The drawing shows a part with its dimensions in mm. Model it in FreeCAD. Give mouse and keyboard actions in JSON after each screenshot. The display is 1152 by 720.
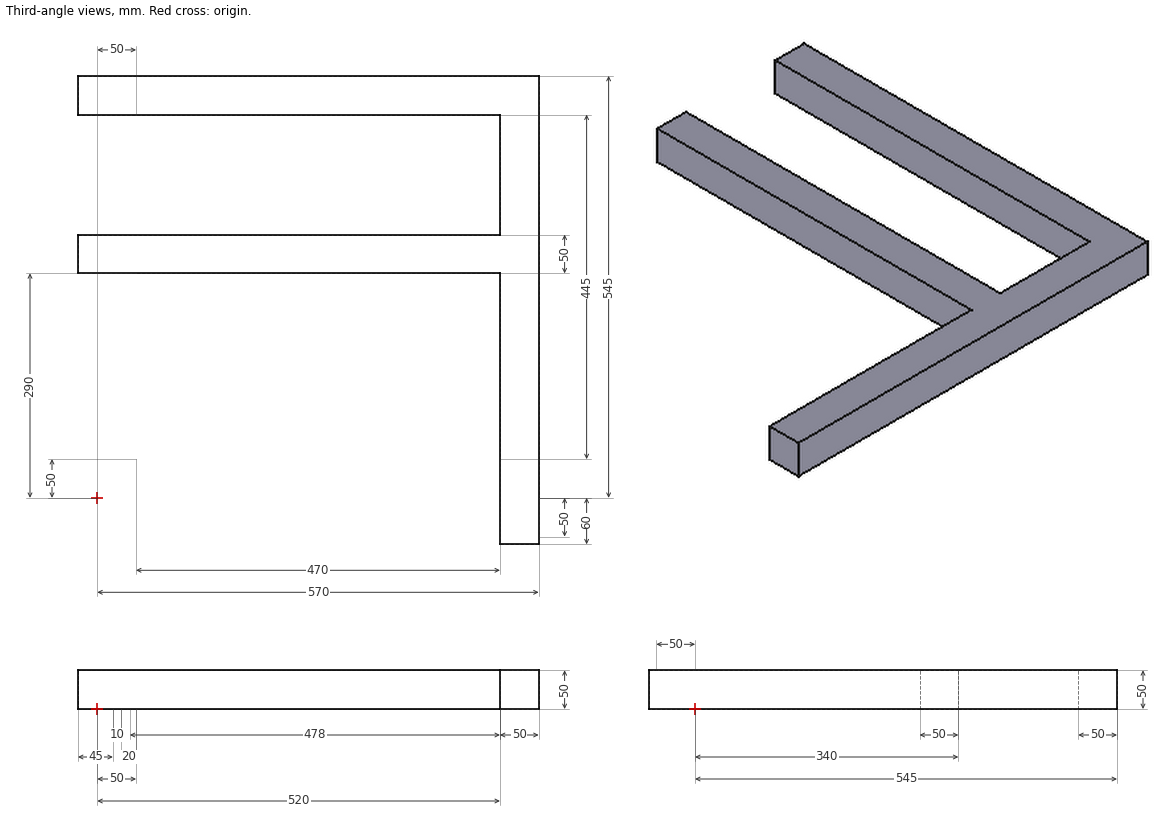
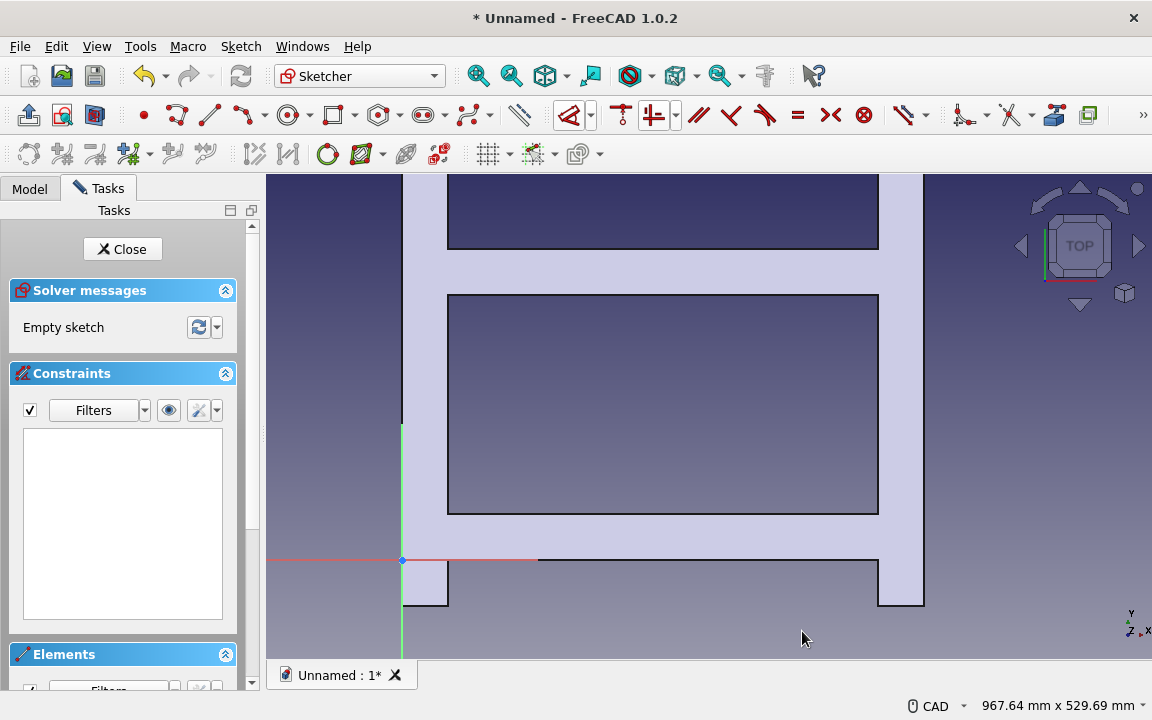
{"action": "left_click", "coordinate": [332, 116]}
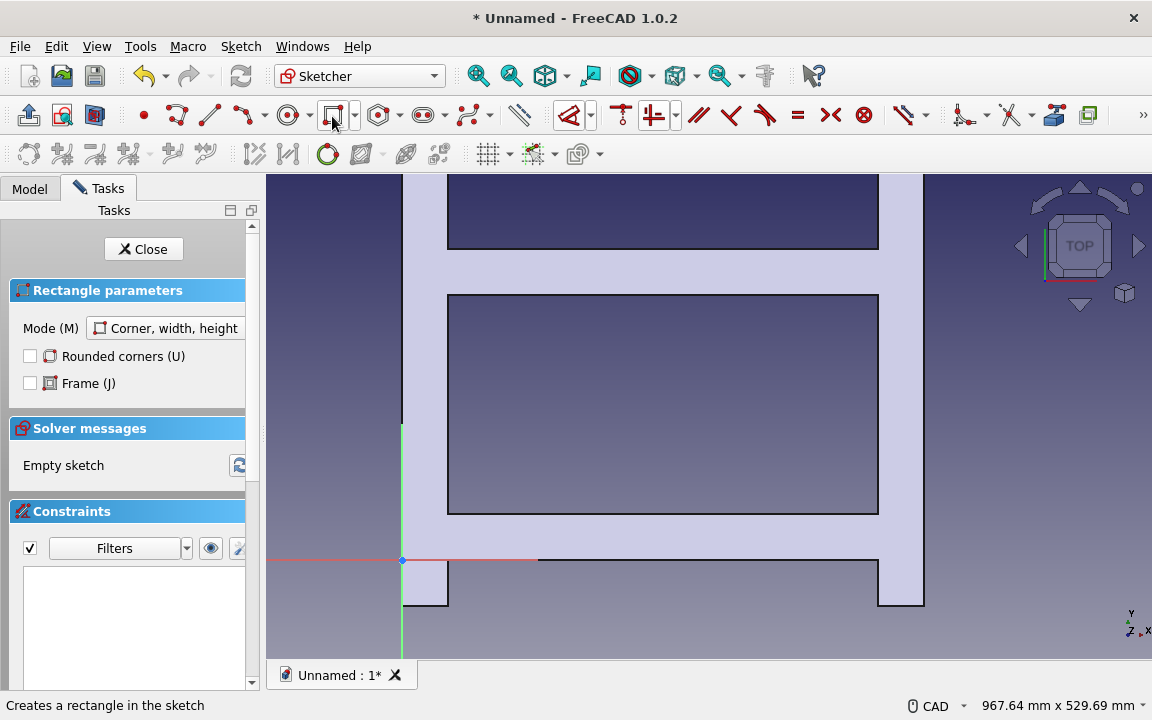
{"action": "left_click", "coordinate": [448, 514]}
{"action": "left_click", "coordinate": [878, 560]}
{"action": "key", "text": "Escape"}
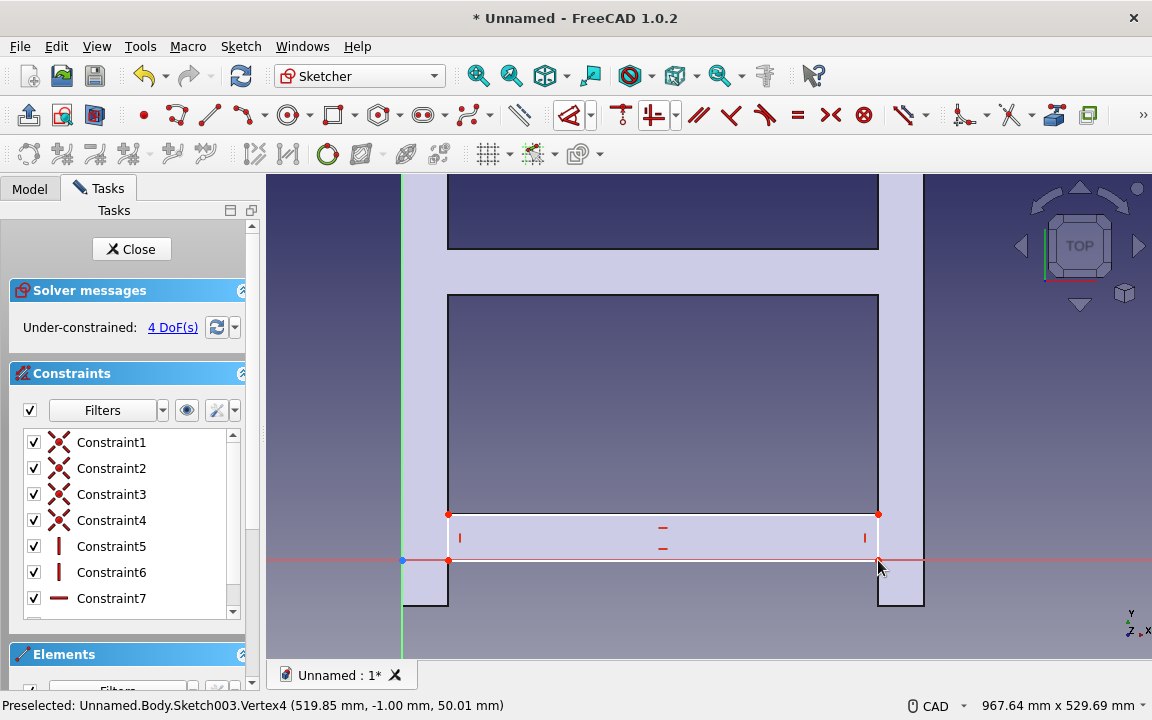
{"action": "left_click", "coordinate": [448, 561]}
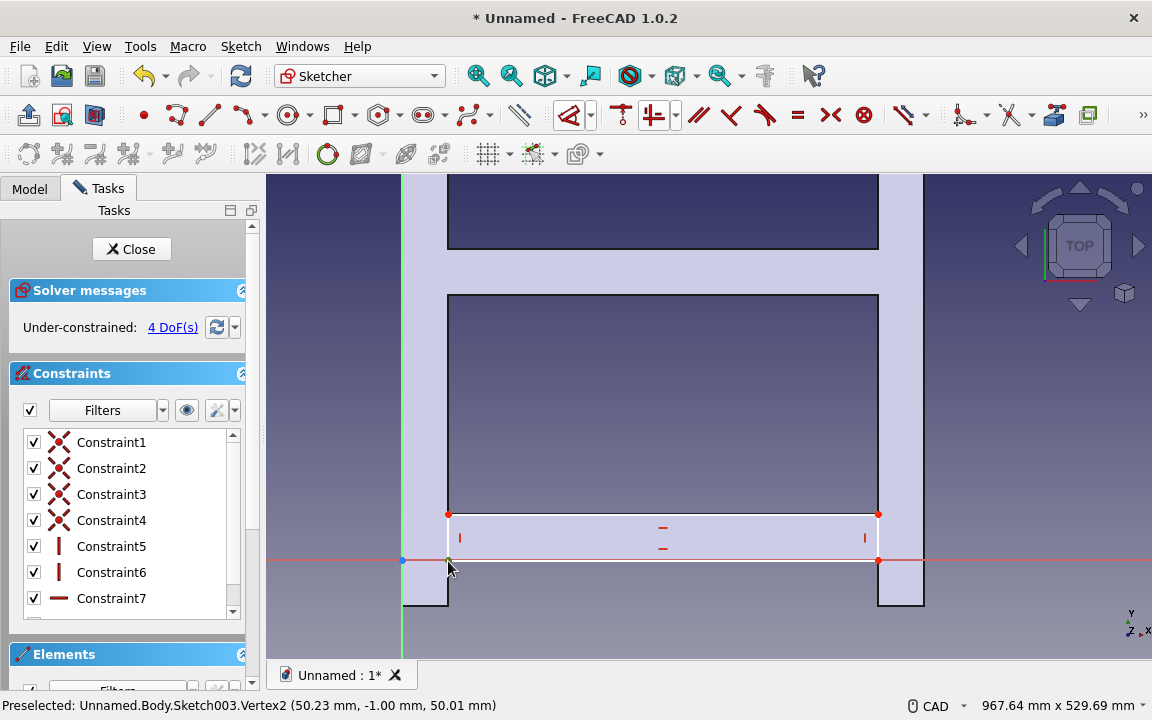
{"action": "left_click", "coordinate": [344, 560]}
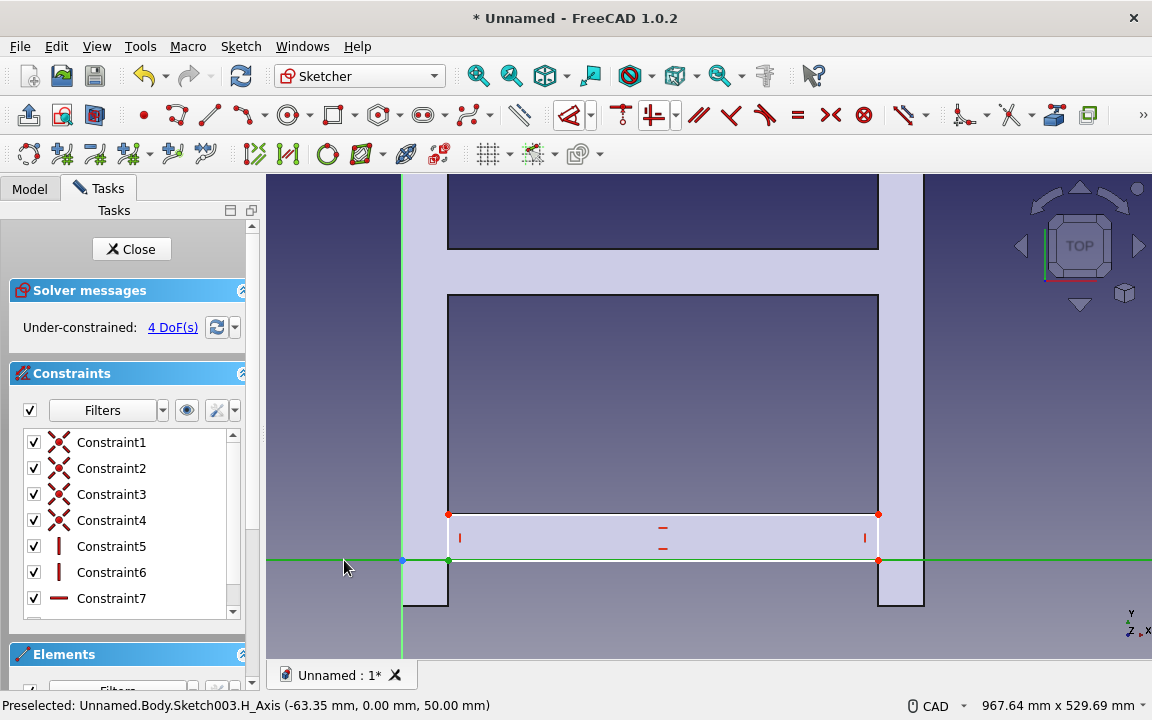
{"action": "key", "text": "c"}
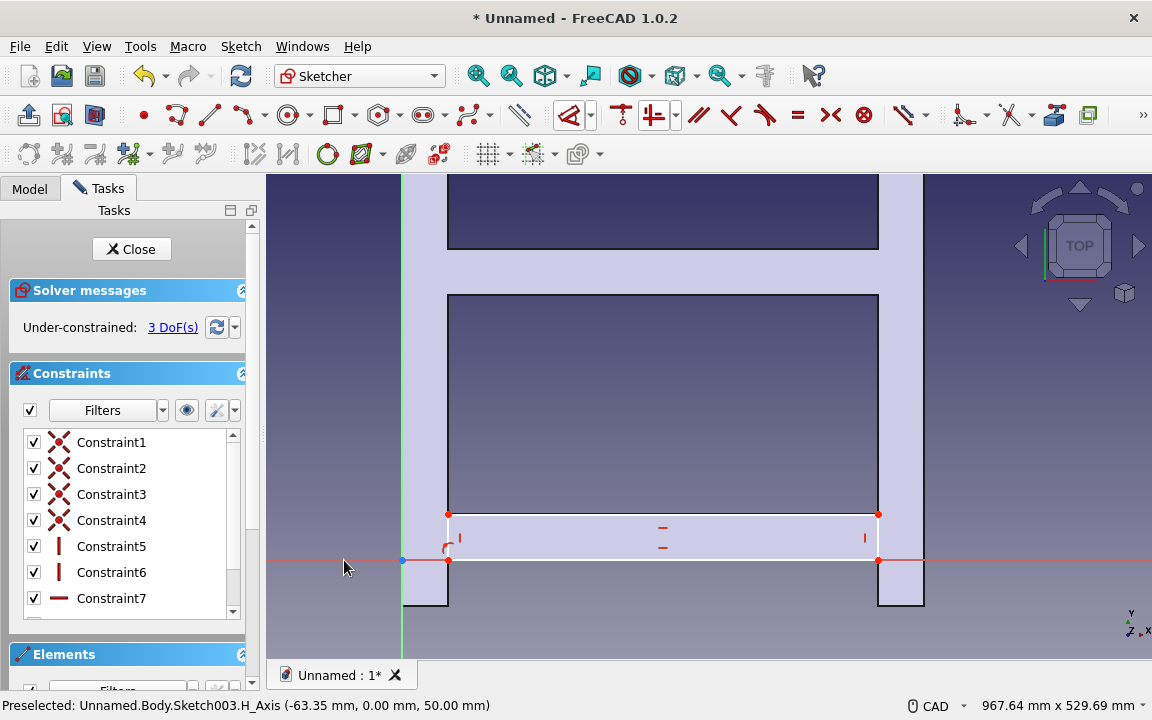
{"action": "left_click", "coordinate": [448, 529]}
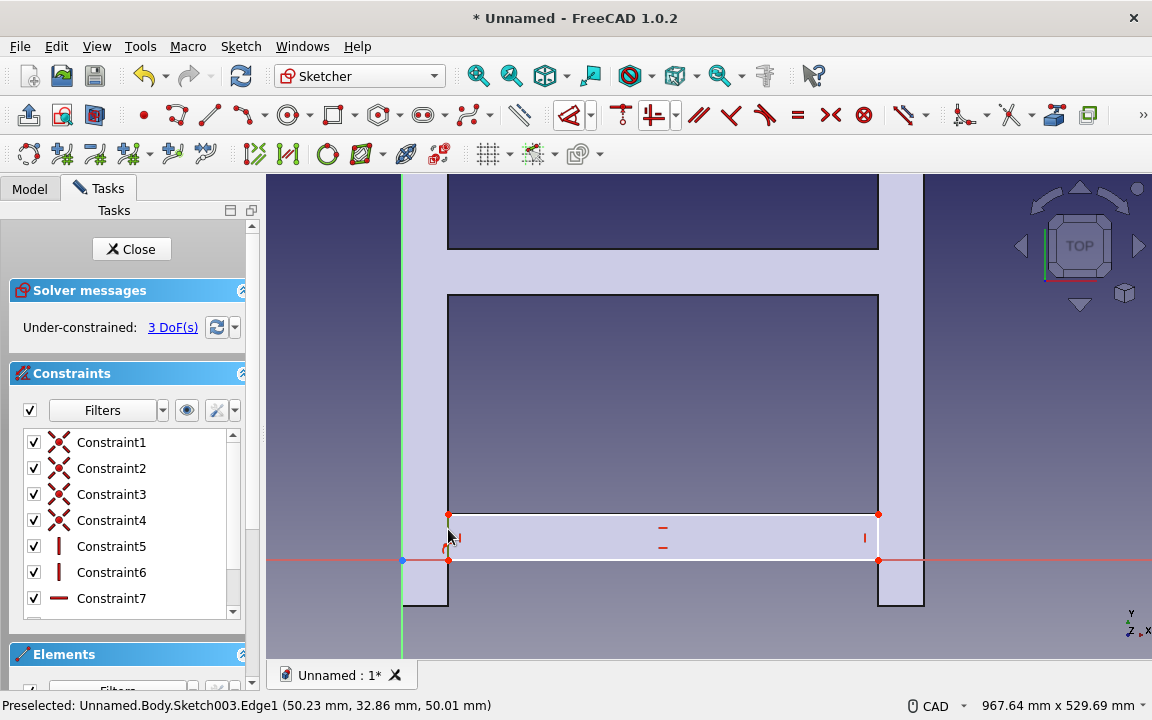
{"action": "key", "text": "i"}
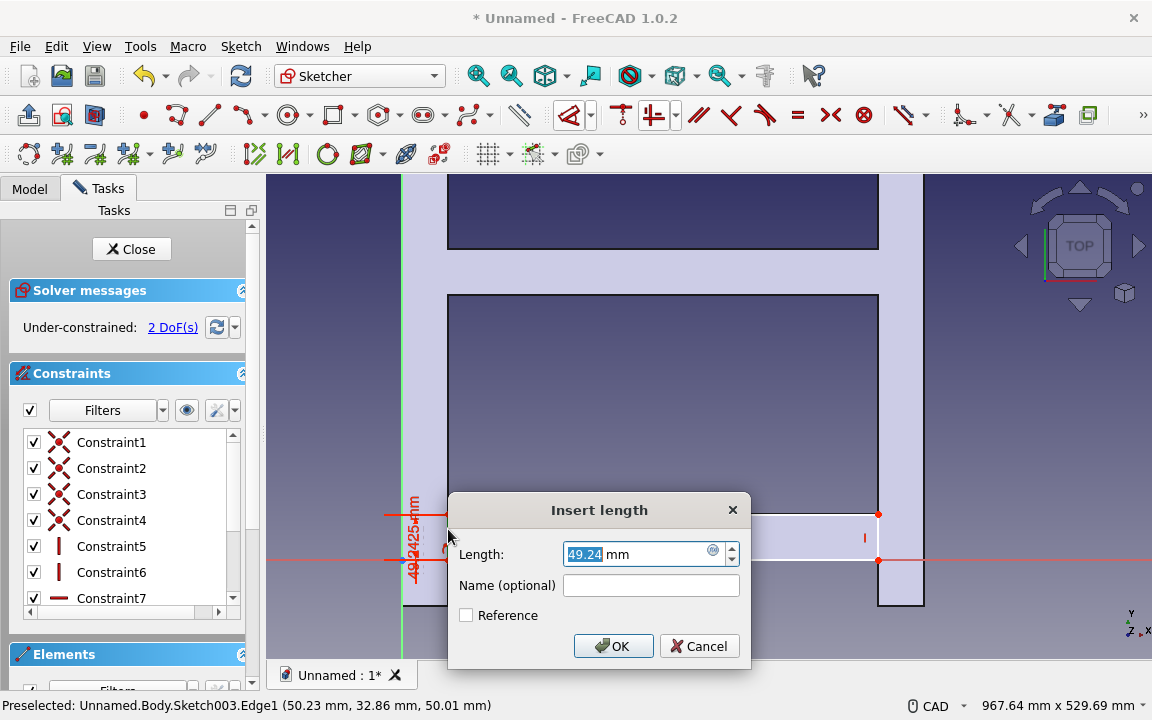
{"action": "type", "text": "50"}
{"action": "key", "text": "Return"}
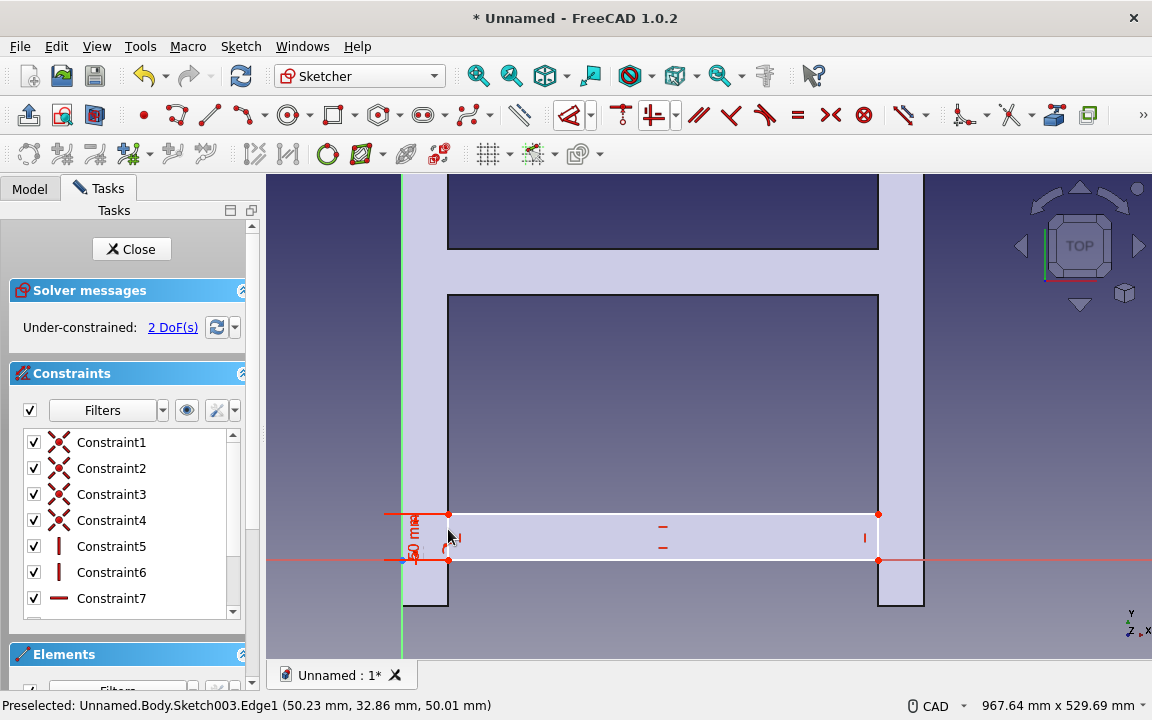
{"action": "left_click", "coordinate": [577, 560]}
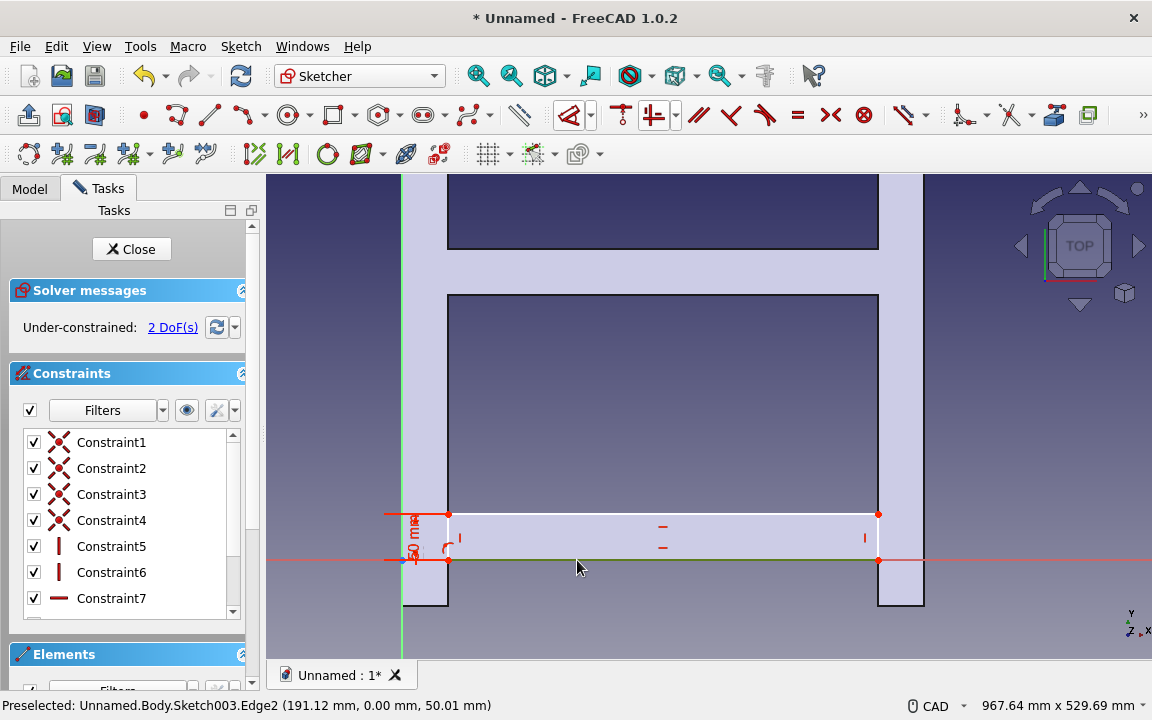
{"action": "key", "text": "l"}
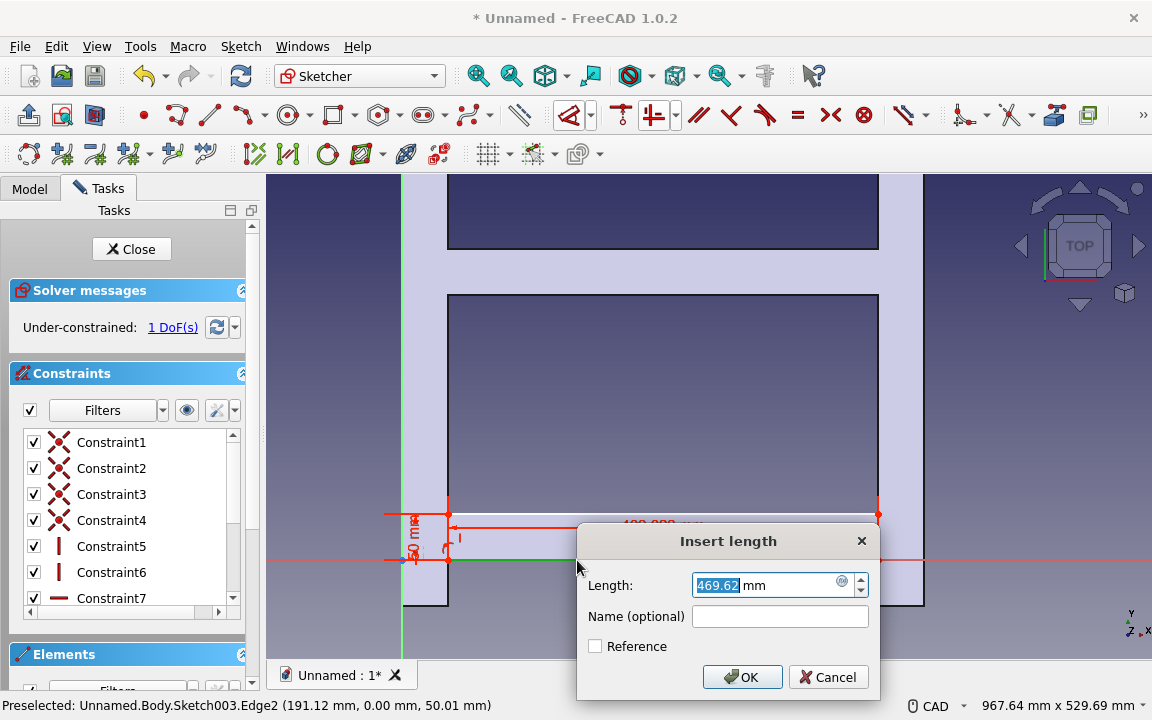
{"action": "type", "text": "470"}
{"action": "key", "text": "Return"}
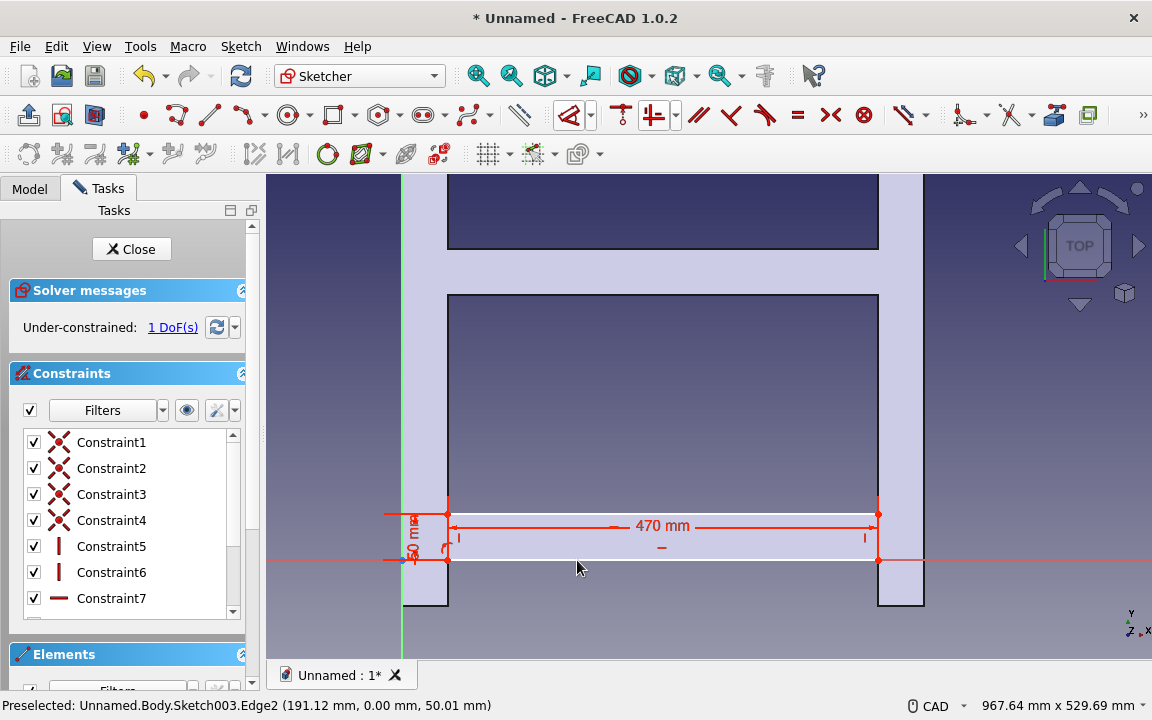
{"action": "left_click", "coordinate": [448, 514]}